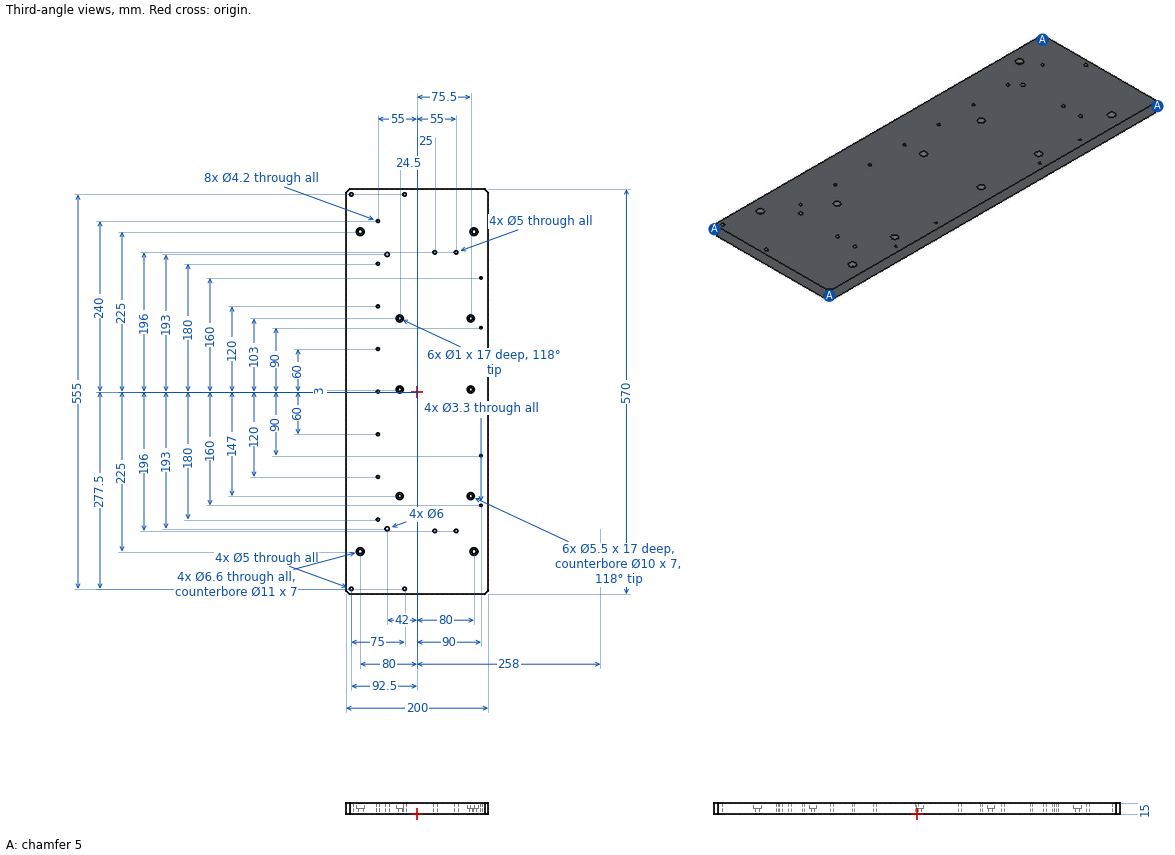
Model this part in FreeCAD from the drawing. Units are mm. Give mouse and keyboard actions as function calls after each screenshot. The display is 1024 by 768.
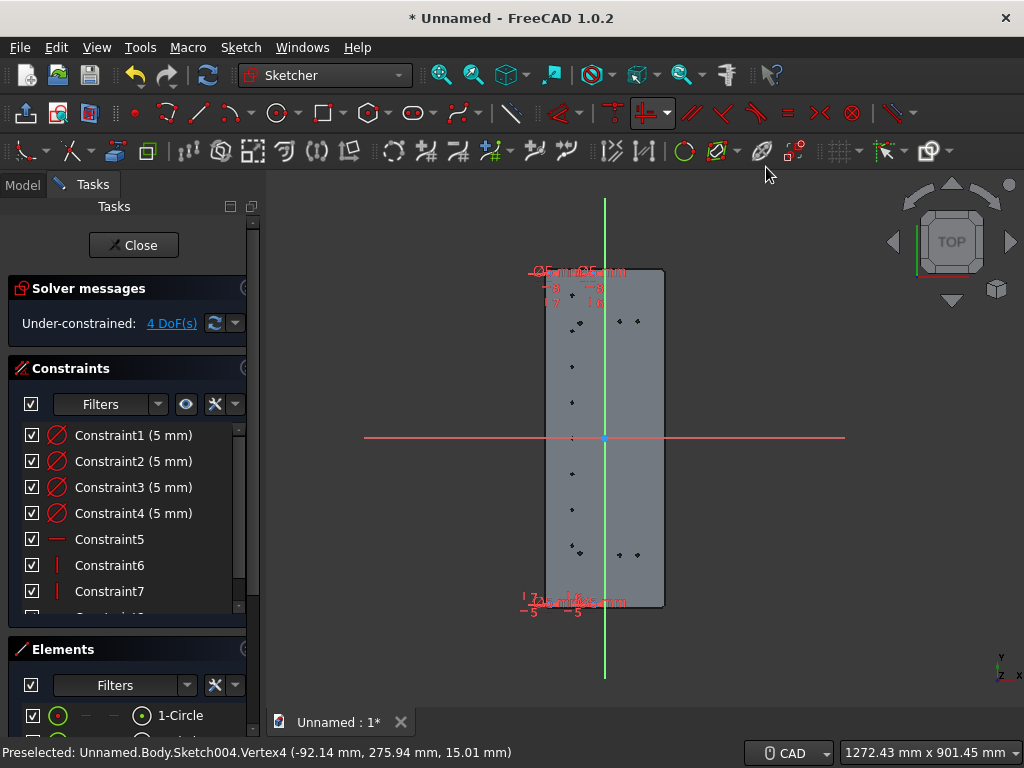
click(558, 114)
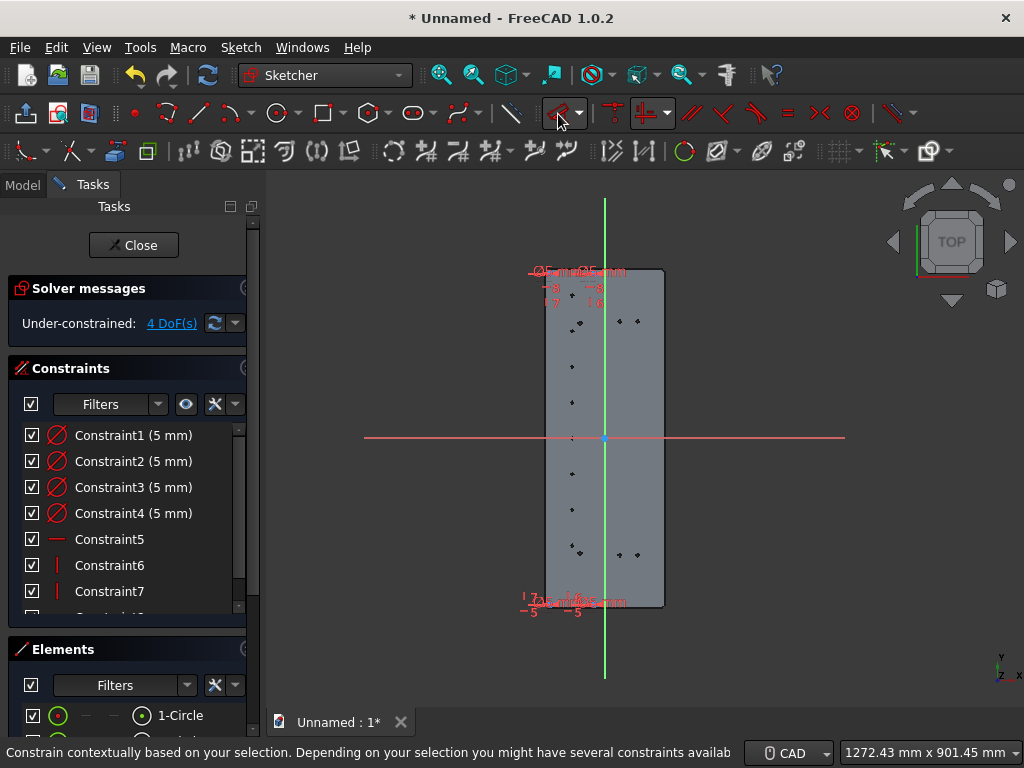
click(550, 605)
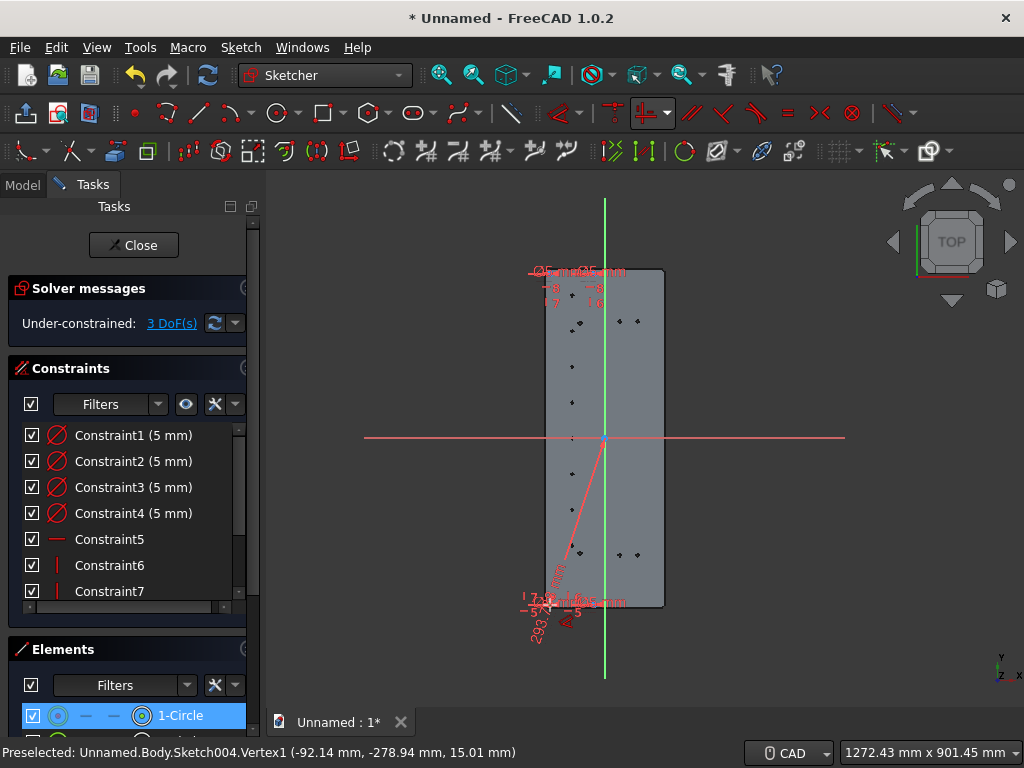
click(594, 605)
click(572, 639)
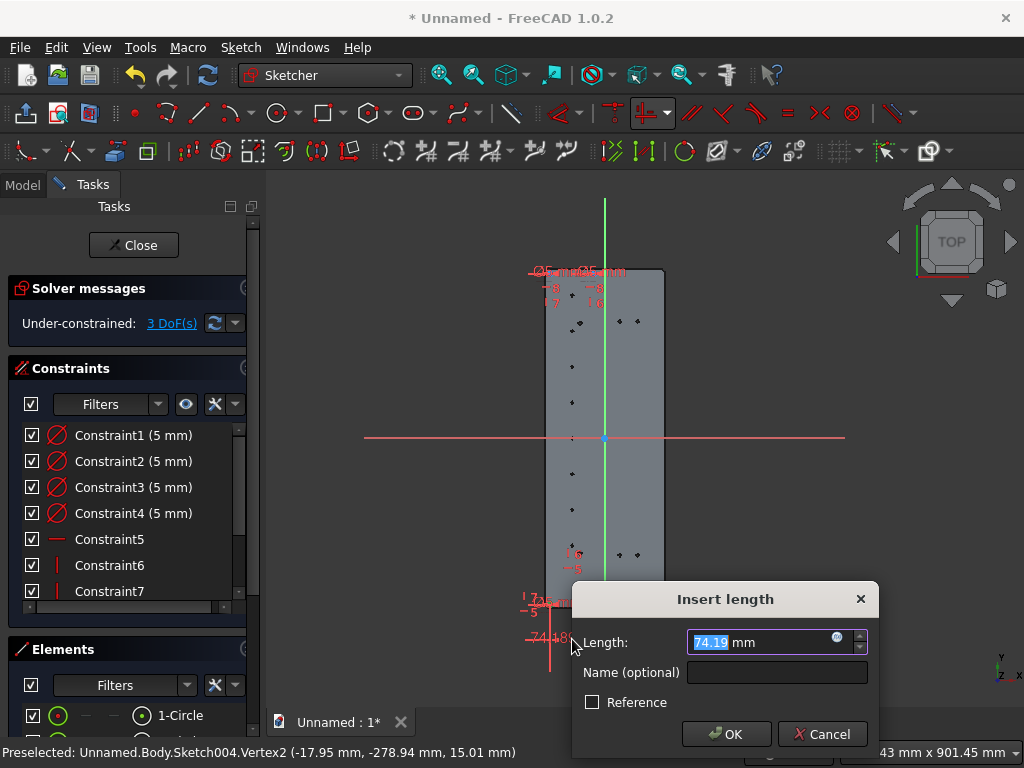
text(75)
key(Return)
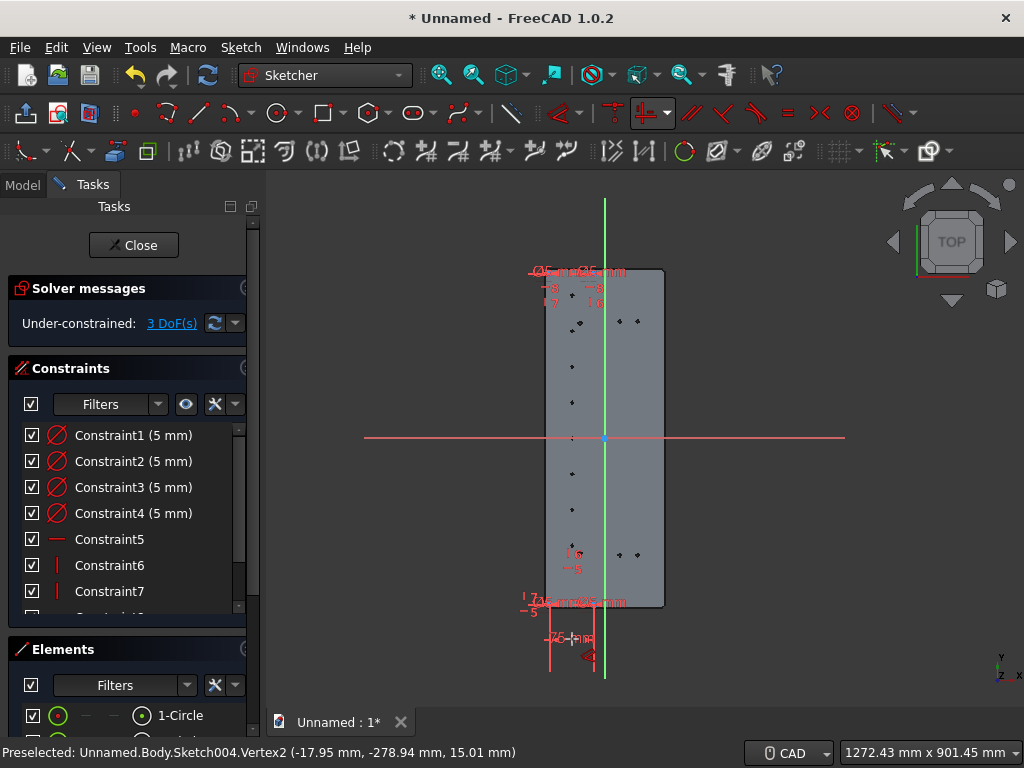
click(550, 605)
click(577, 404)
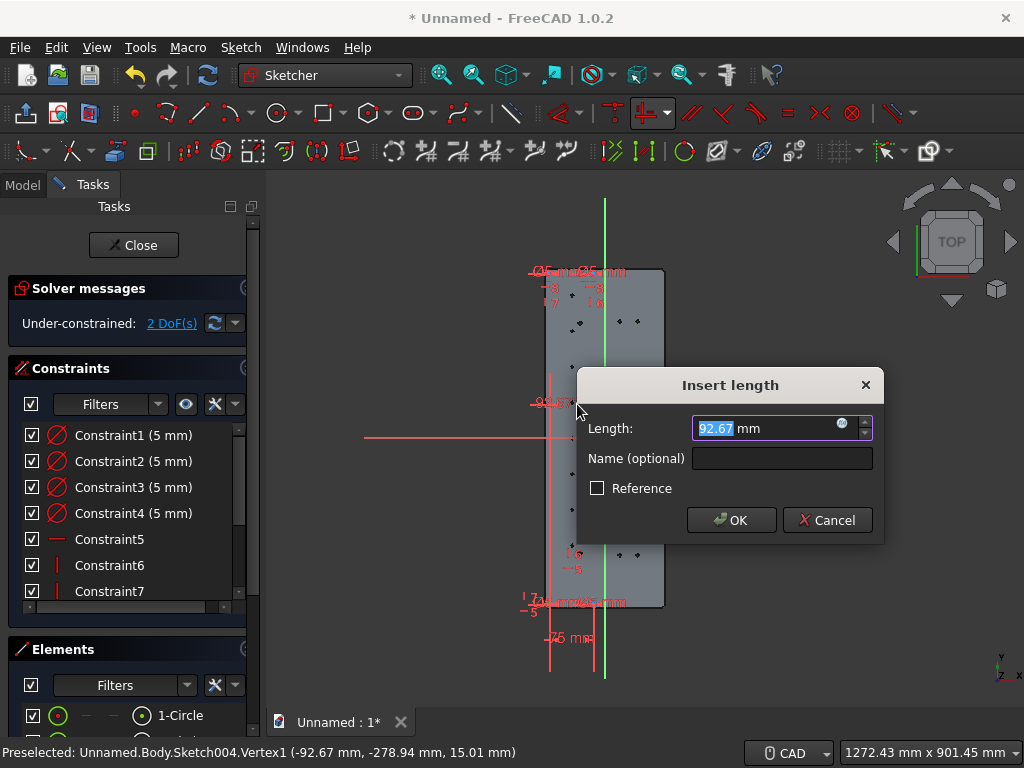
text(92.5)
key(Return)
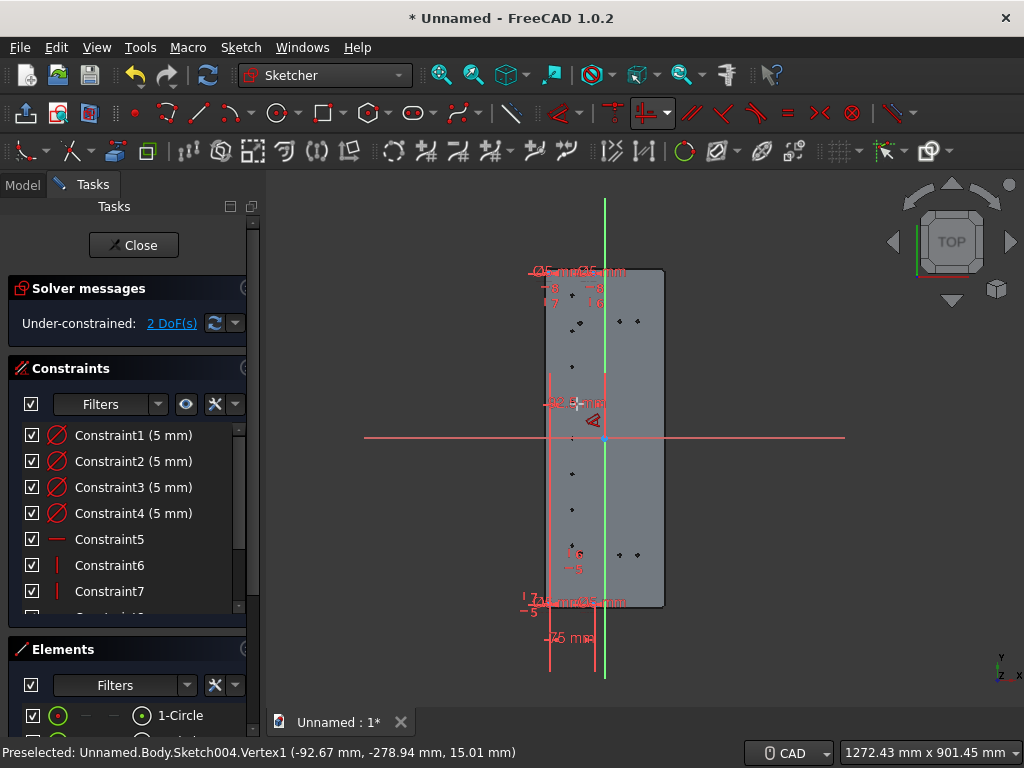
click(595, 605)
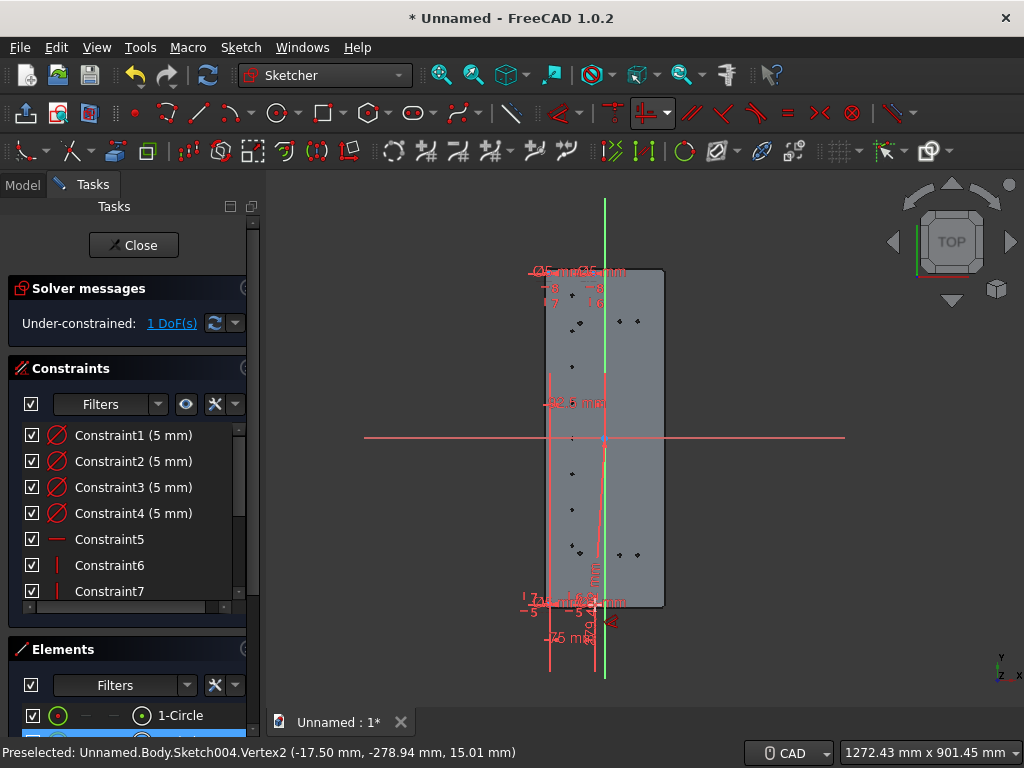
click(595, 274)
click(629, 363)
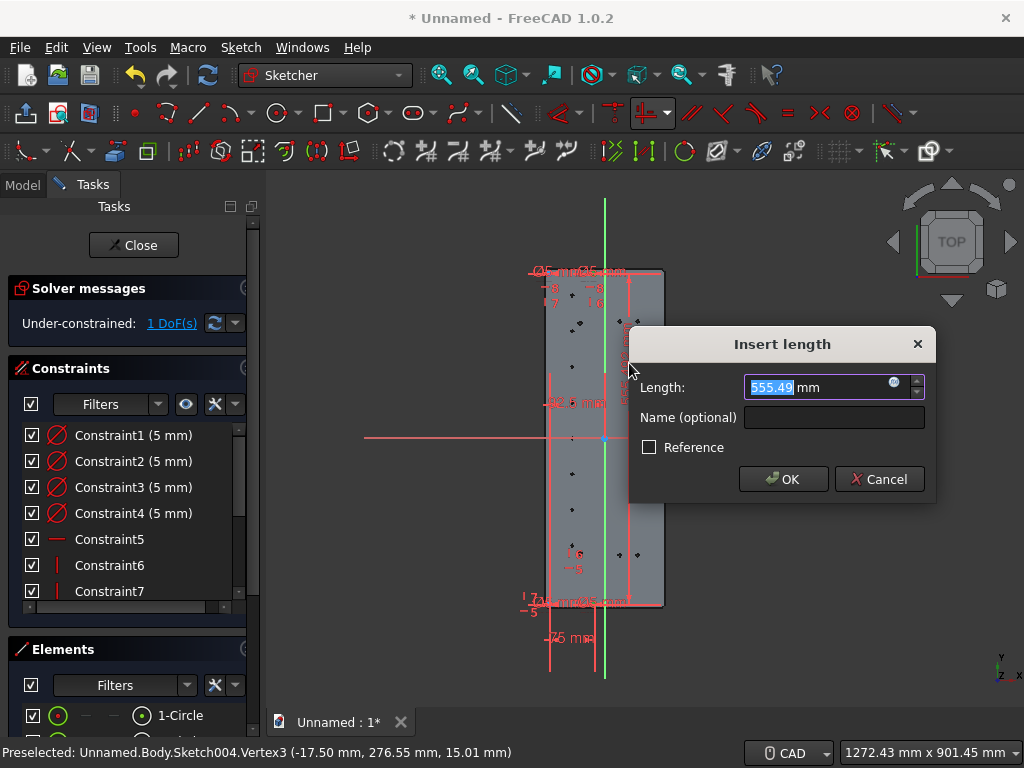
text(555)
key(Return)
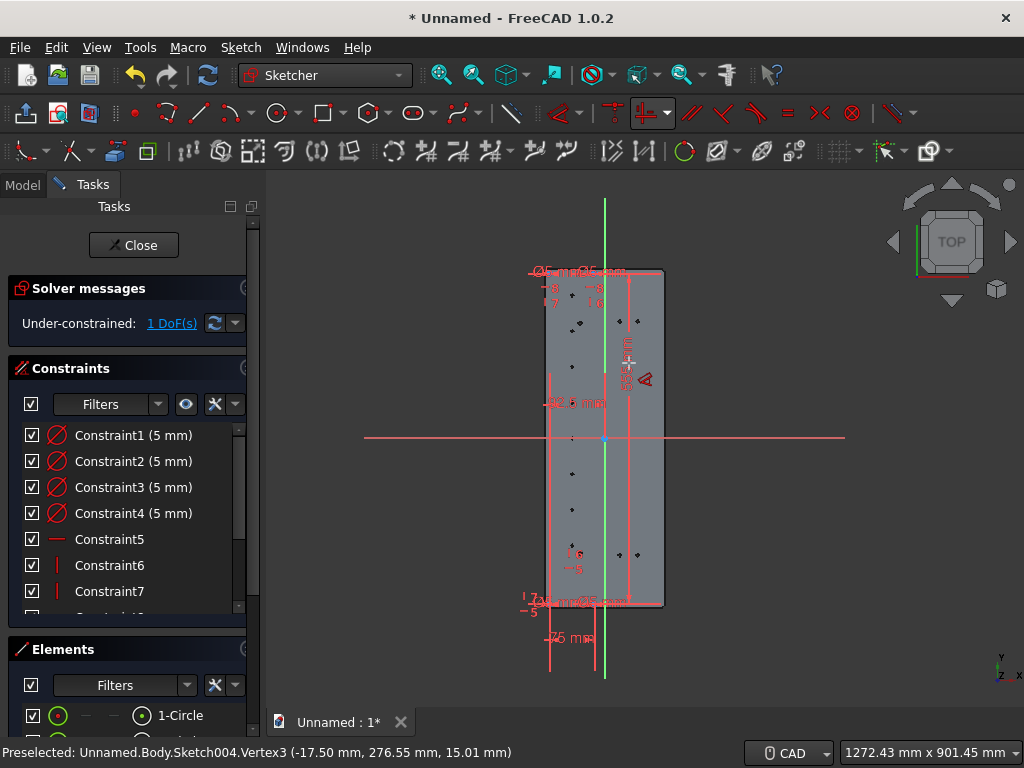
click(550, 604)
click(639, 521)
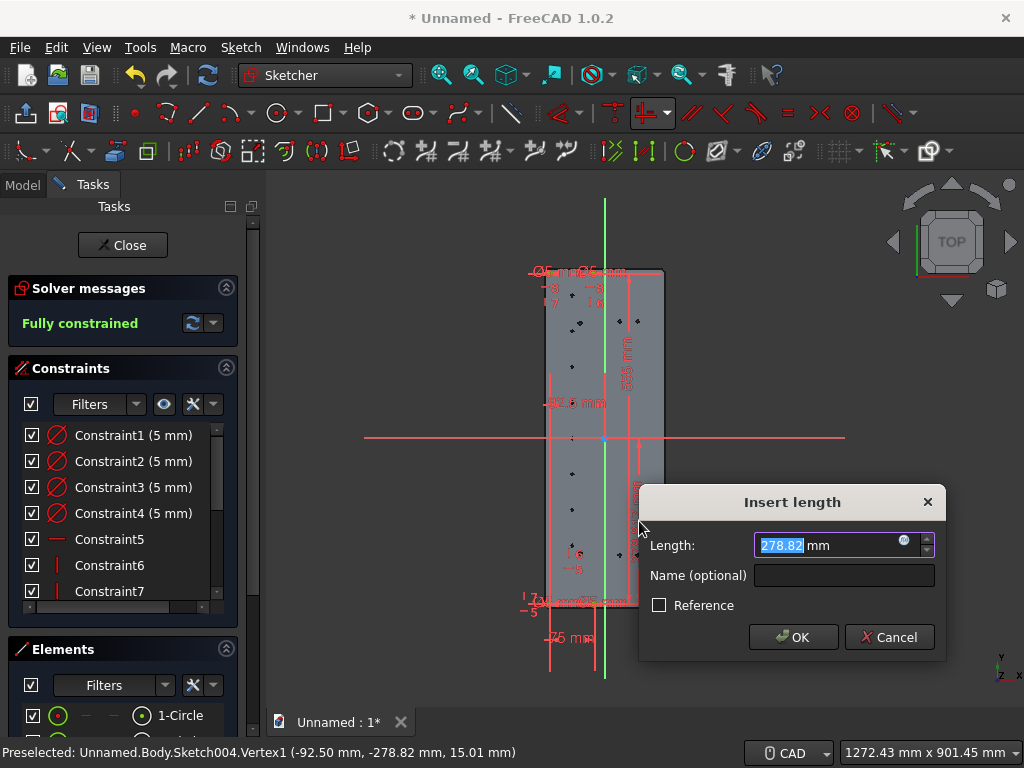
text(277.5)
key(Return)
key(Escape)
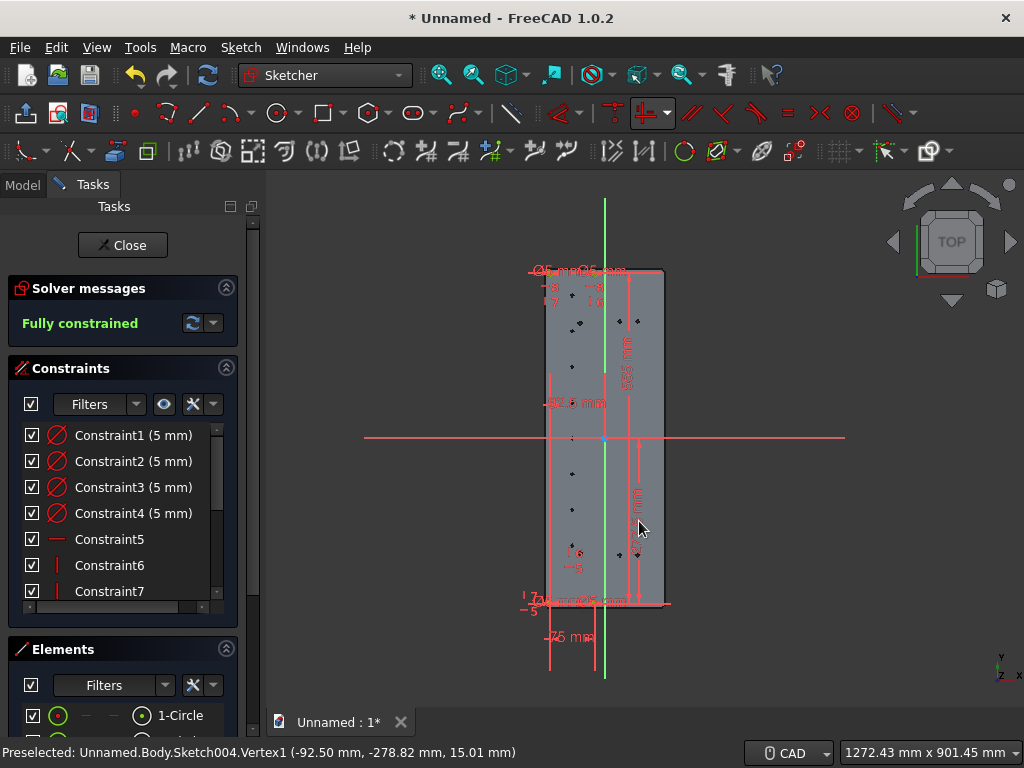
click(123, 245)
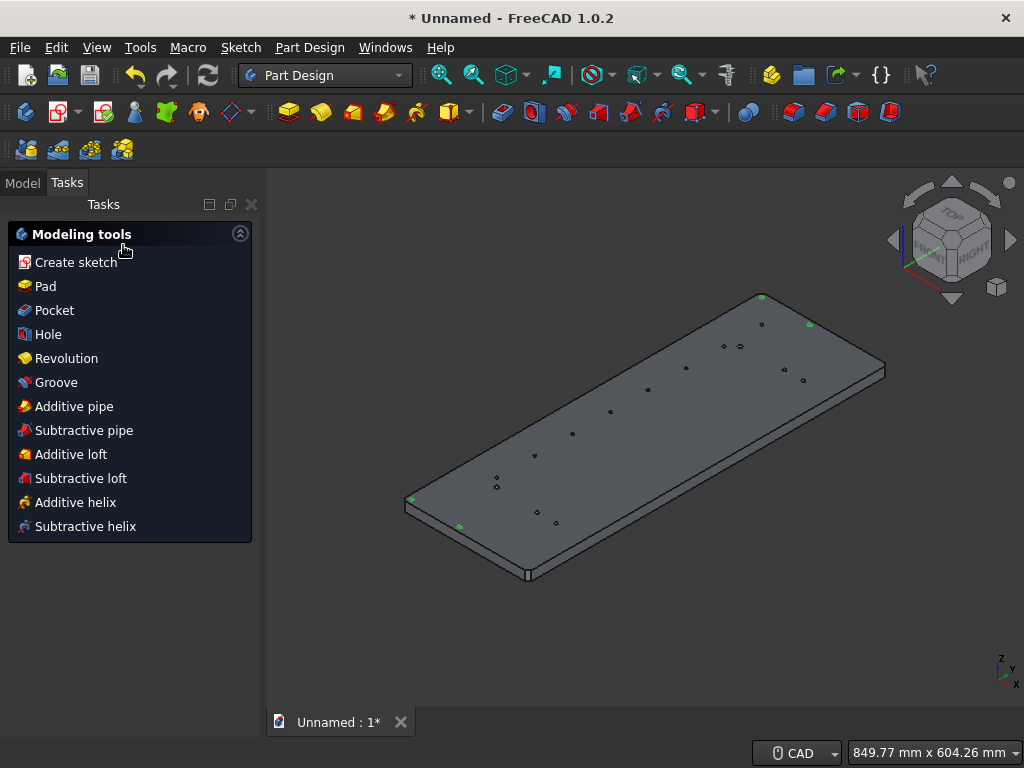
click(536, 112)